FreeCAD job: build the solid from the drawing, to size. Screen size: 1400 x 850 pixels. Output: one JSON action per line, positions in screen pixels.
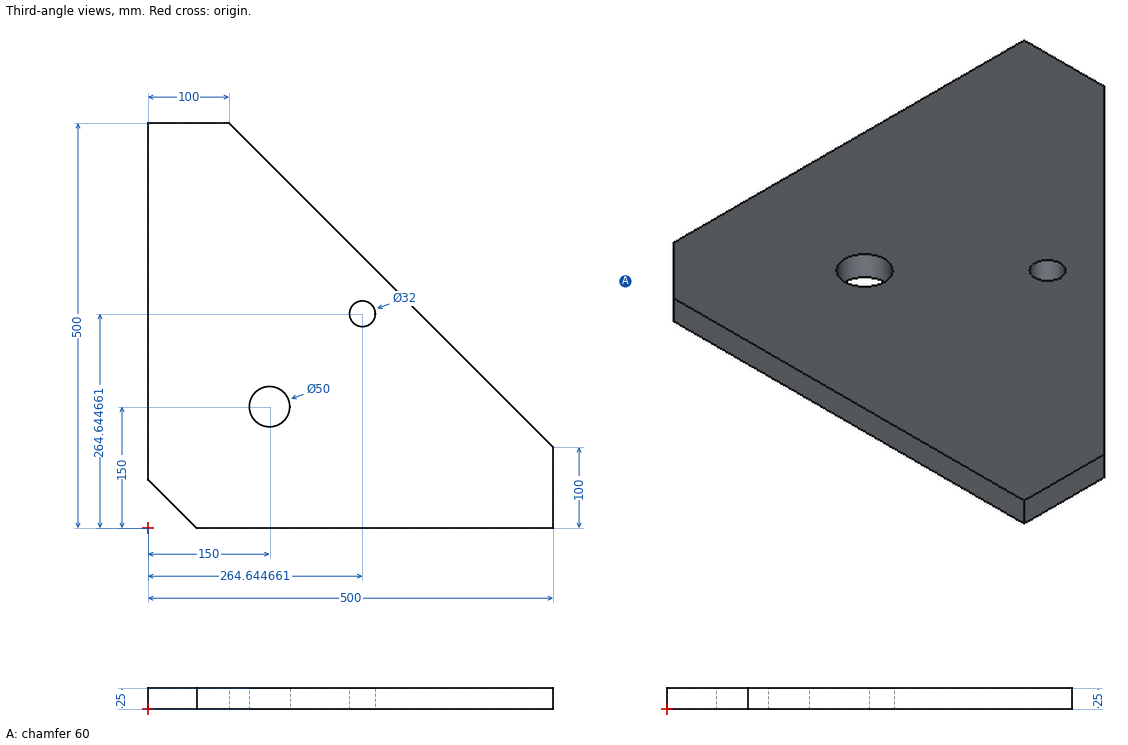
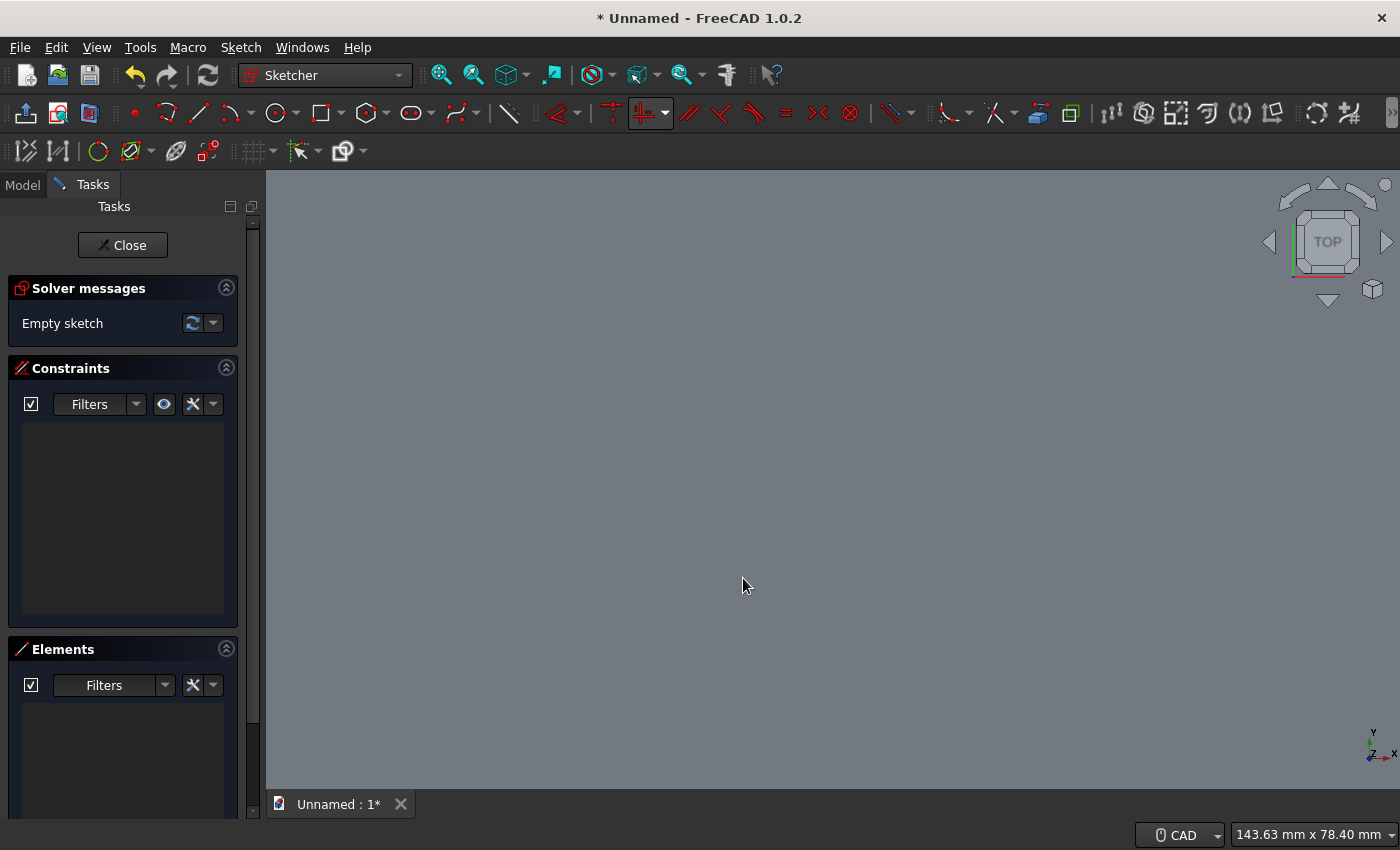
{"action": "left_click", "coordinate": [276, 114]}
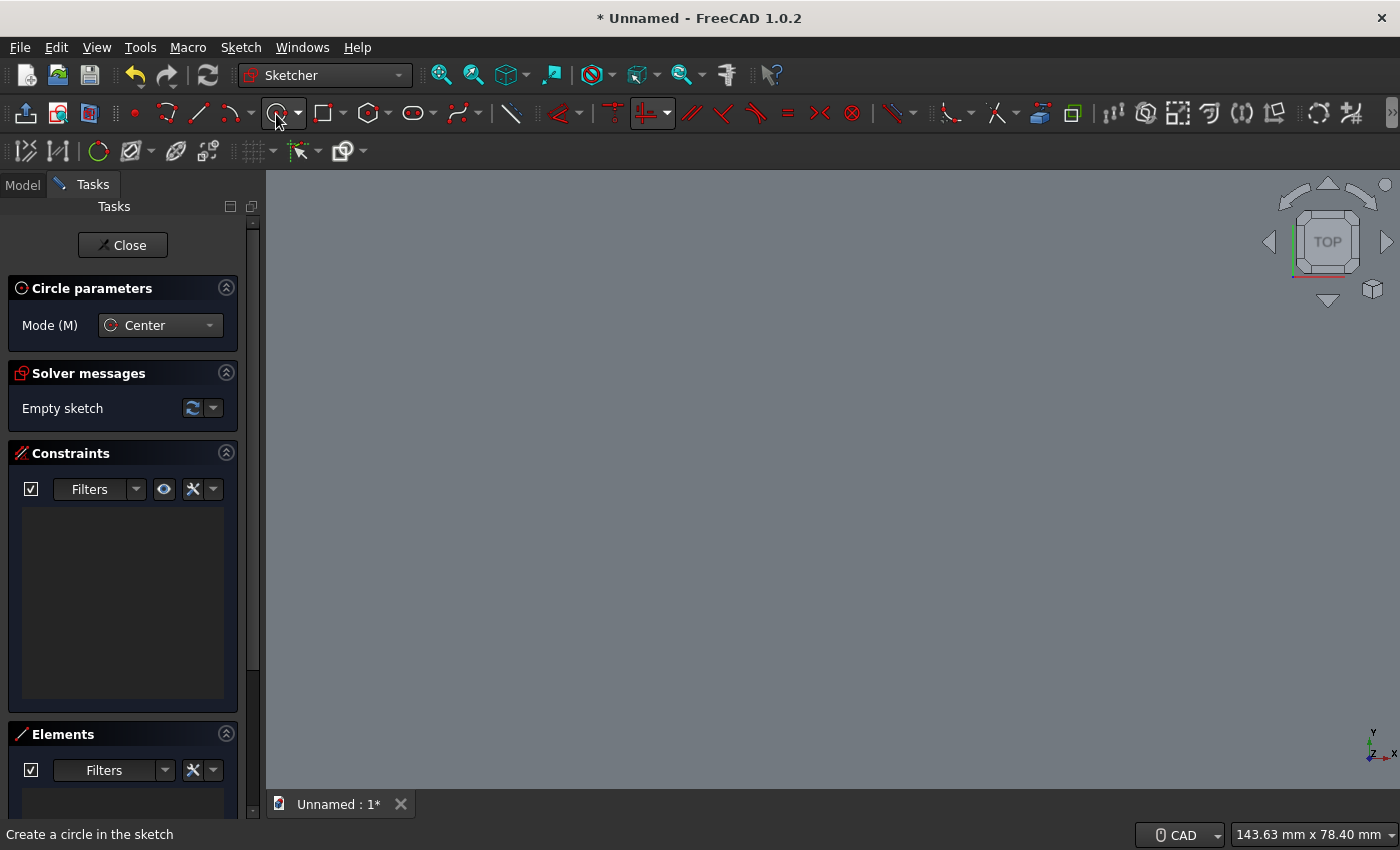
{"action": "left_click", "coordinate": [762, 473]}
{"action": "left_click", "coordinate": [902, 334]}
{"action": "key", "text": "Escape"}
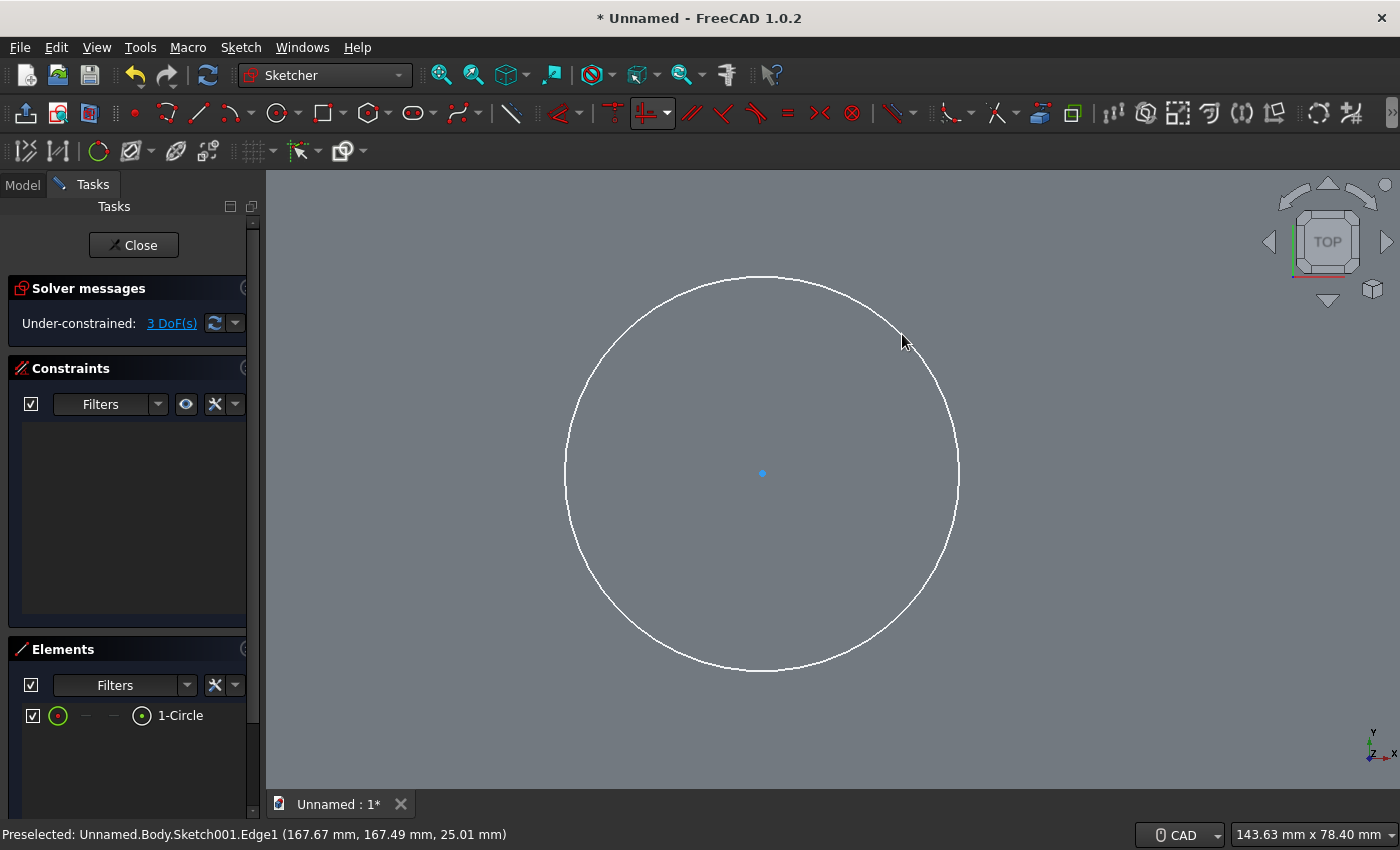
{"action": "left_click", "coordinate": [558, 114]}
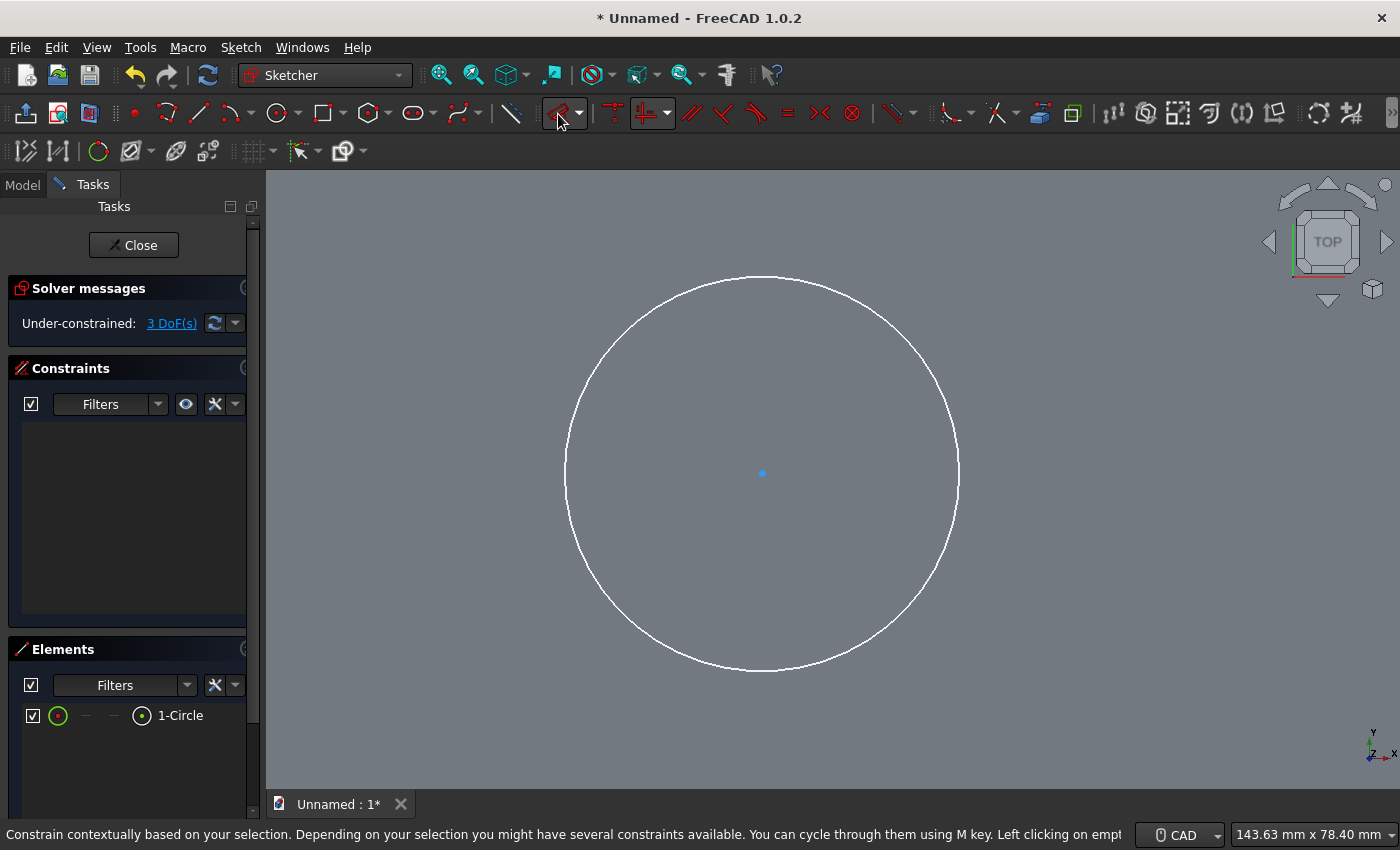
{"action": "left_click", "coordinate": [901, 334]}
{"action": "left_click", "coordinate": [924, 311]}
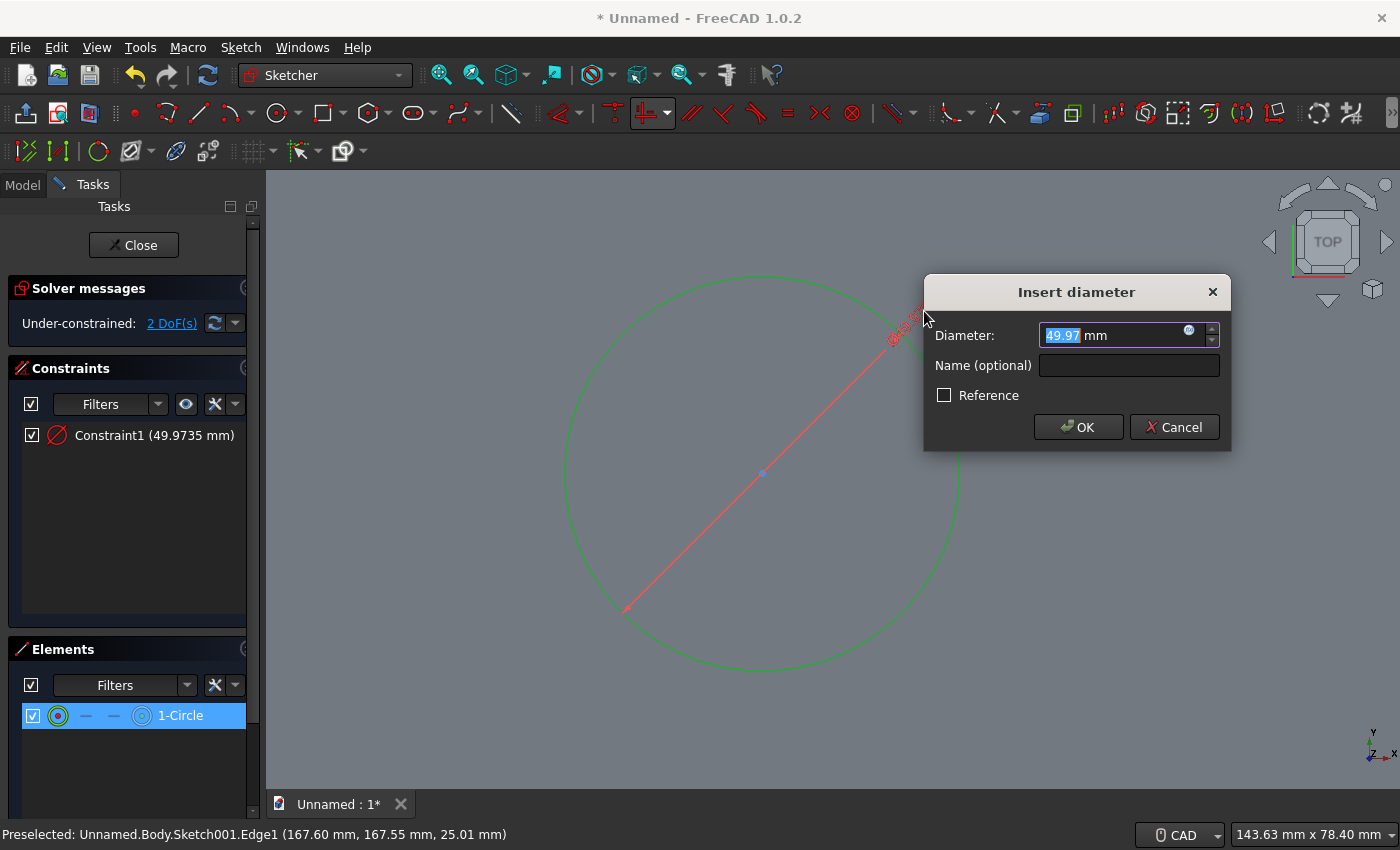
{"action": "type", "text": "50"}
{"action": "key", "text": "Return"}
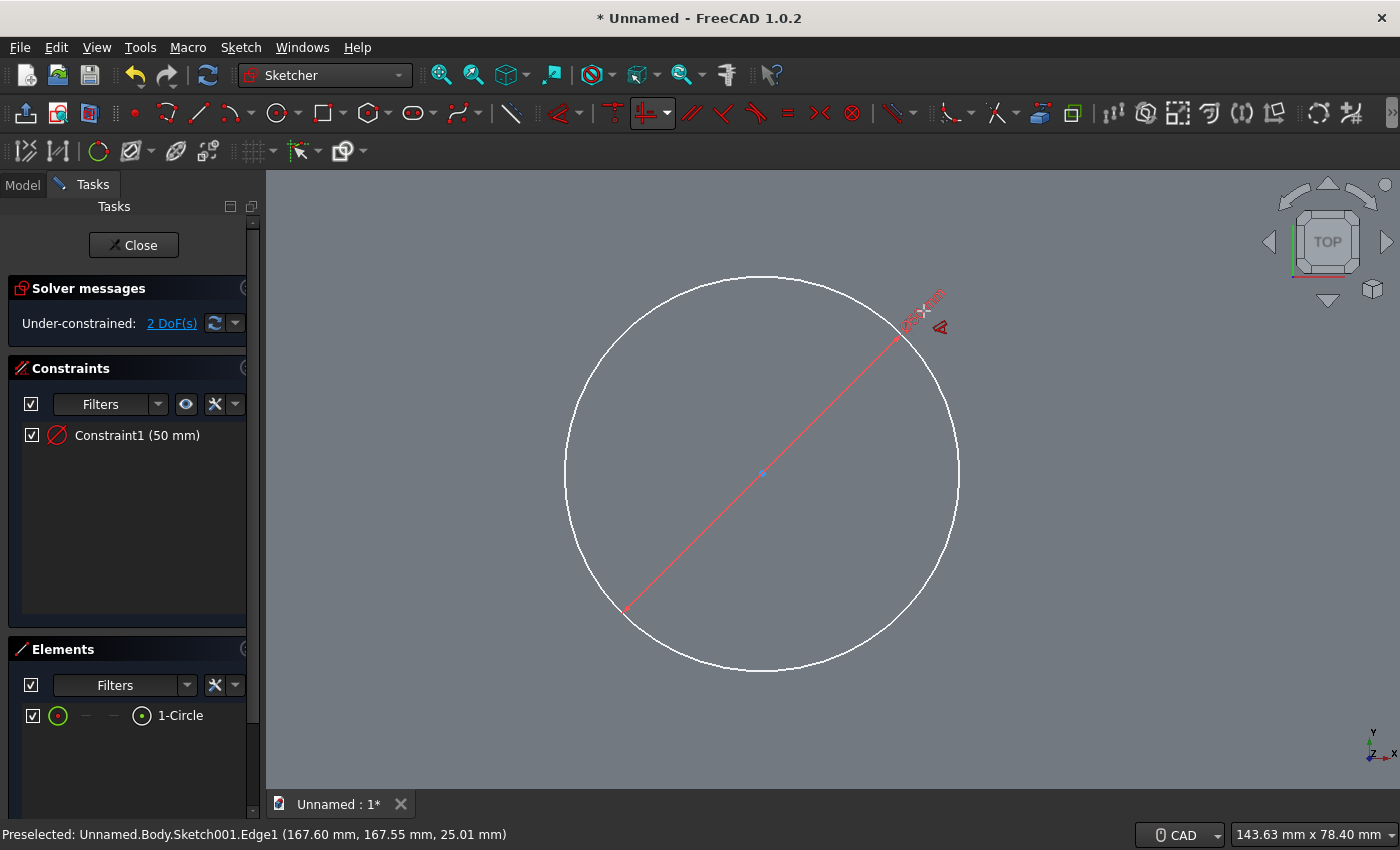
{"action": "left_click", "coordinate": [762, 474]}
{"action": "left_click", "coordinate": [528, 440]}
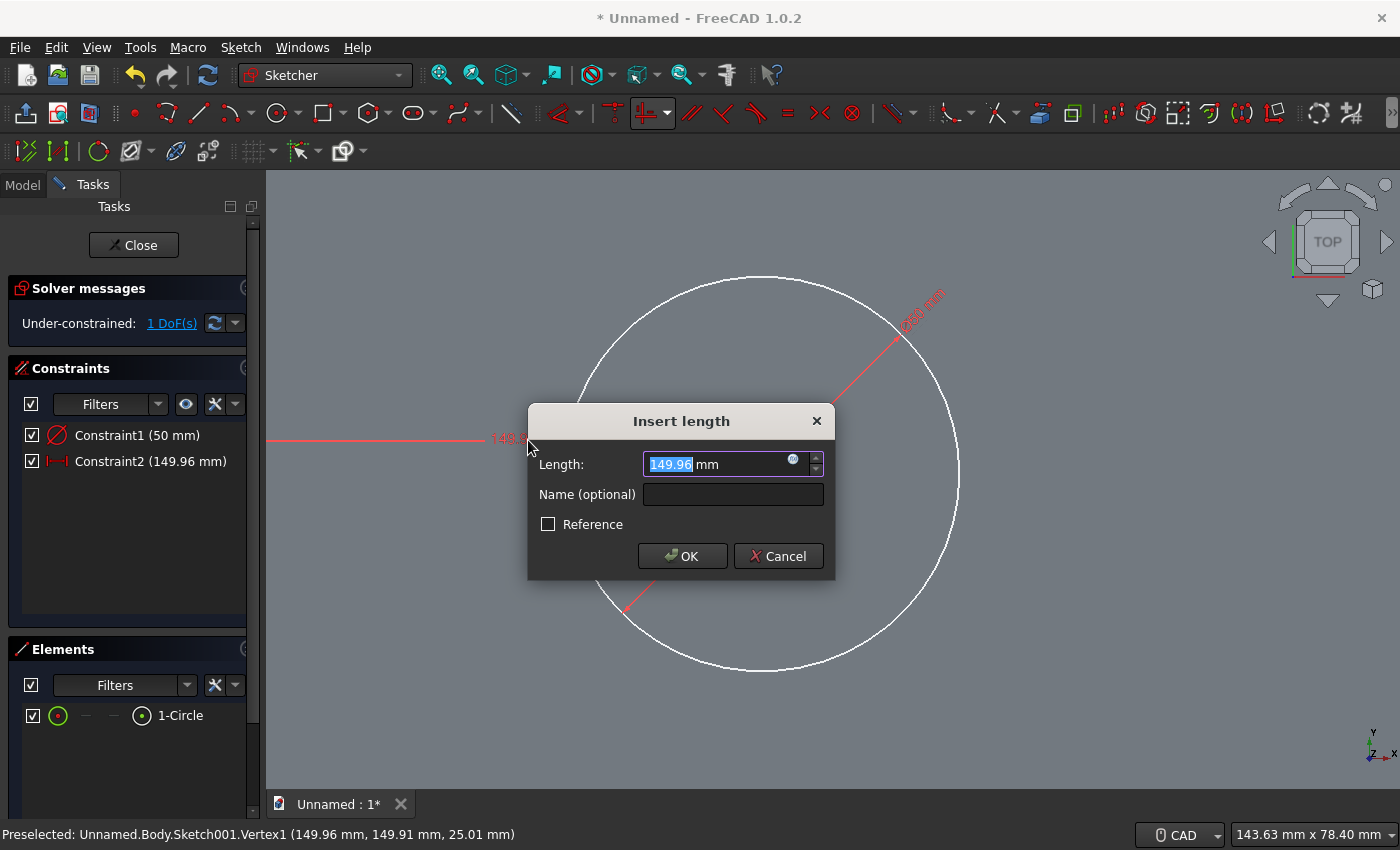
{"action": "type", "text": "150"}
{"action": "key", "text": "Return"}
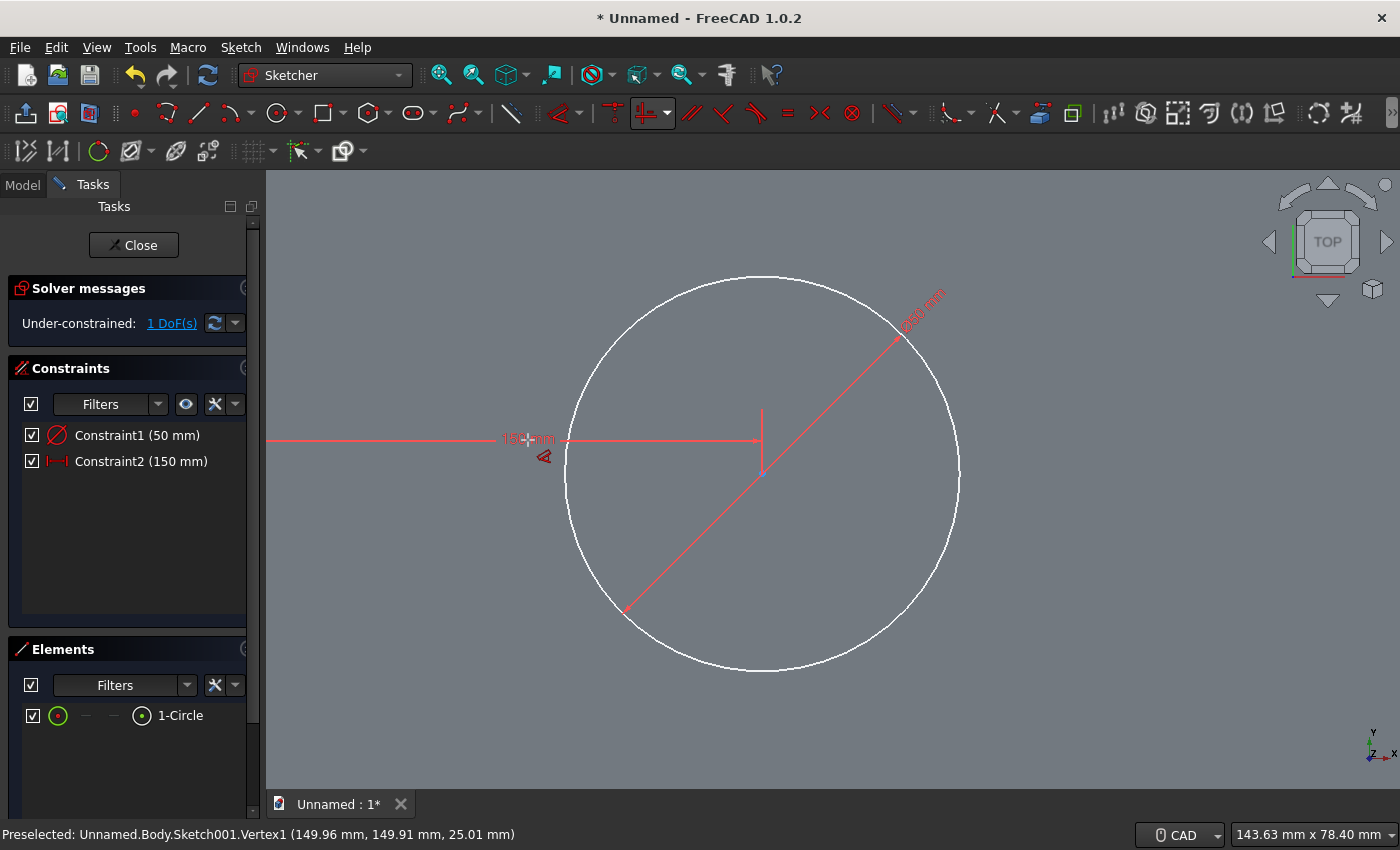
{"action": "left_click", "coordinate": [762, 474]}
{"action": "left_click", "coordinate": [796, 618]}